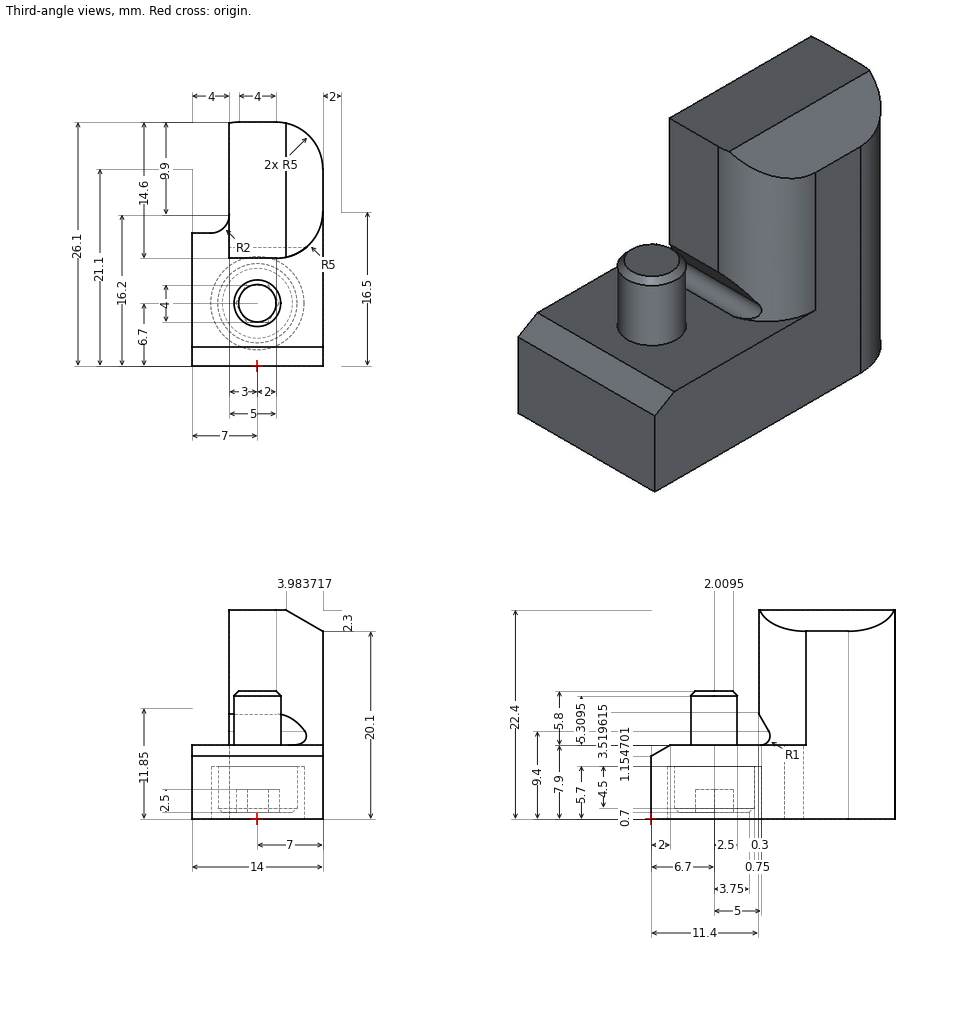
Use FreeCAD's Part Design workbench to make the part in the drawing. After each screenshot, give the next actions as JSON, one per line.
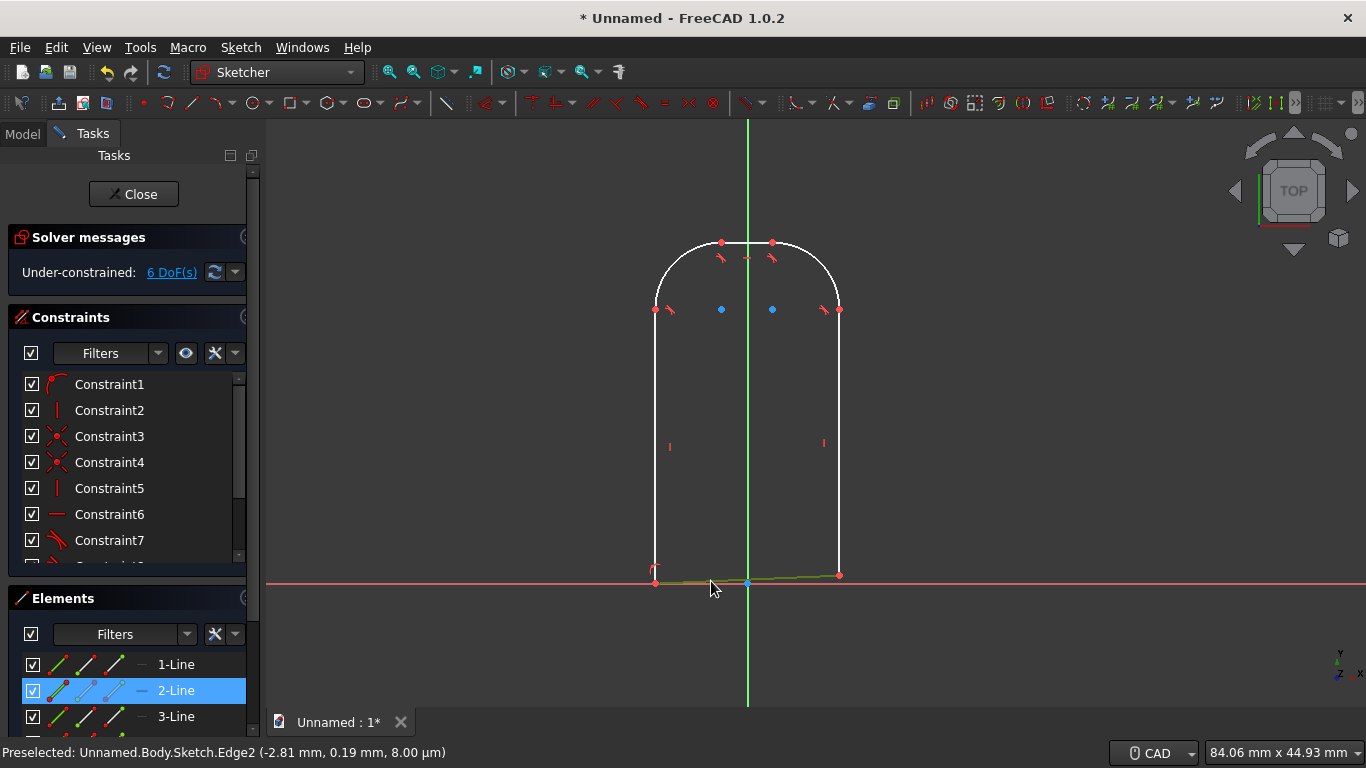
{"action": "key", "text": "h"}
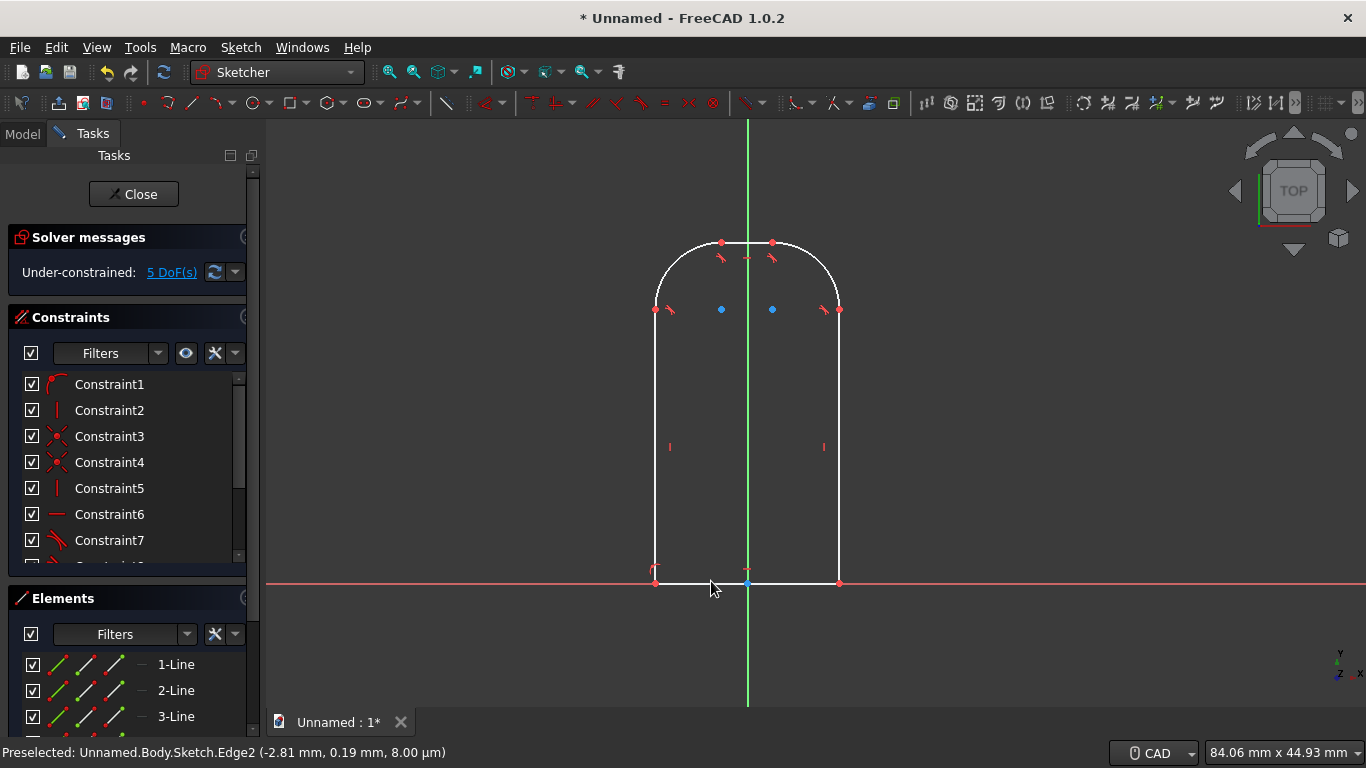
{"action": "left_click", "coordinate": [832, 279]}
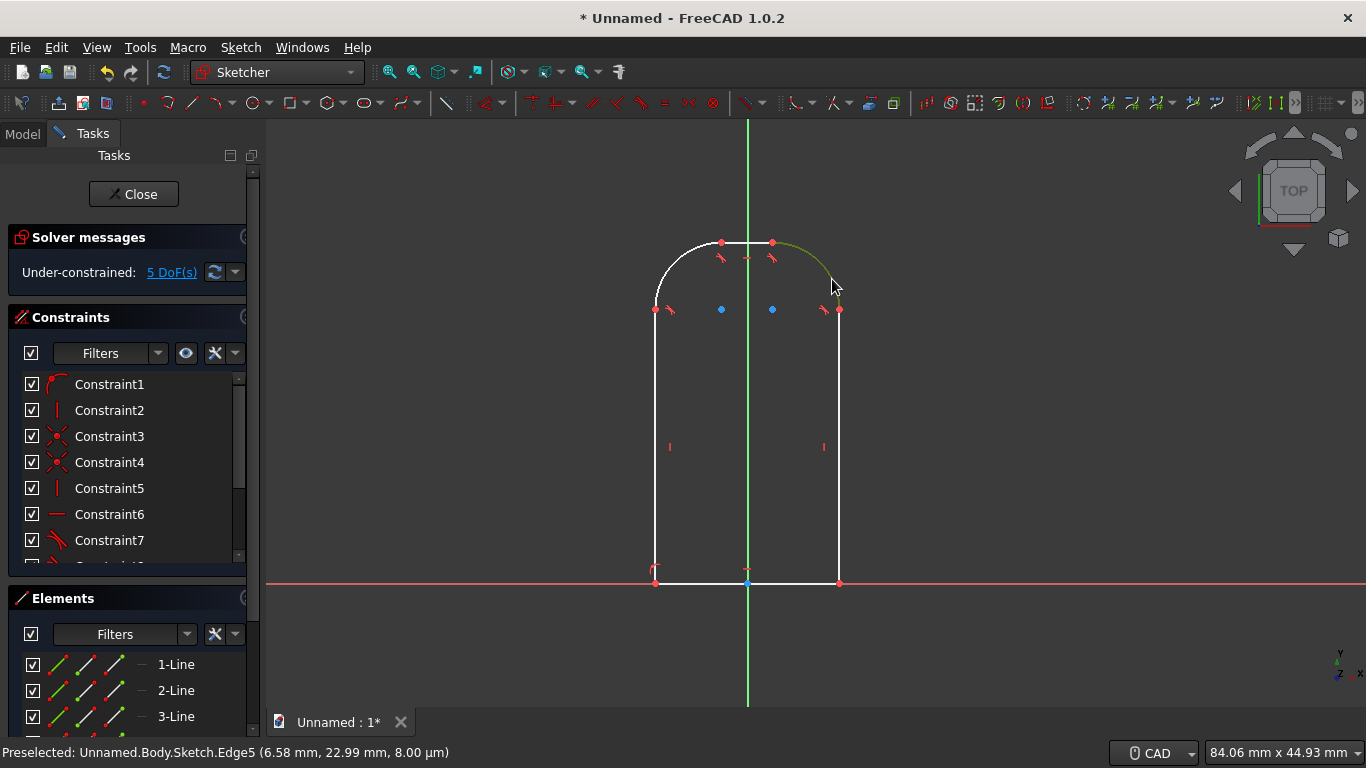
{"action": "left_click", "coordinate": [692, 250]}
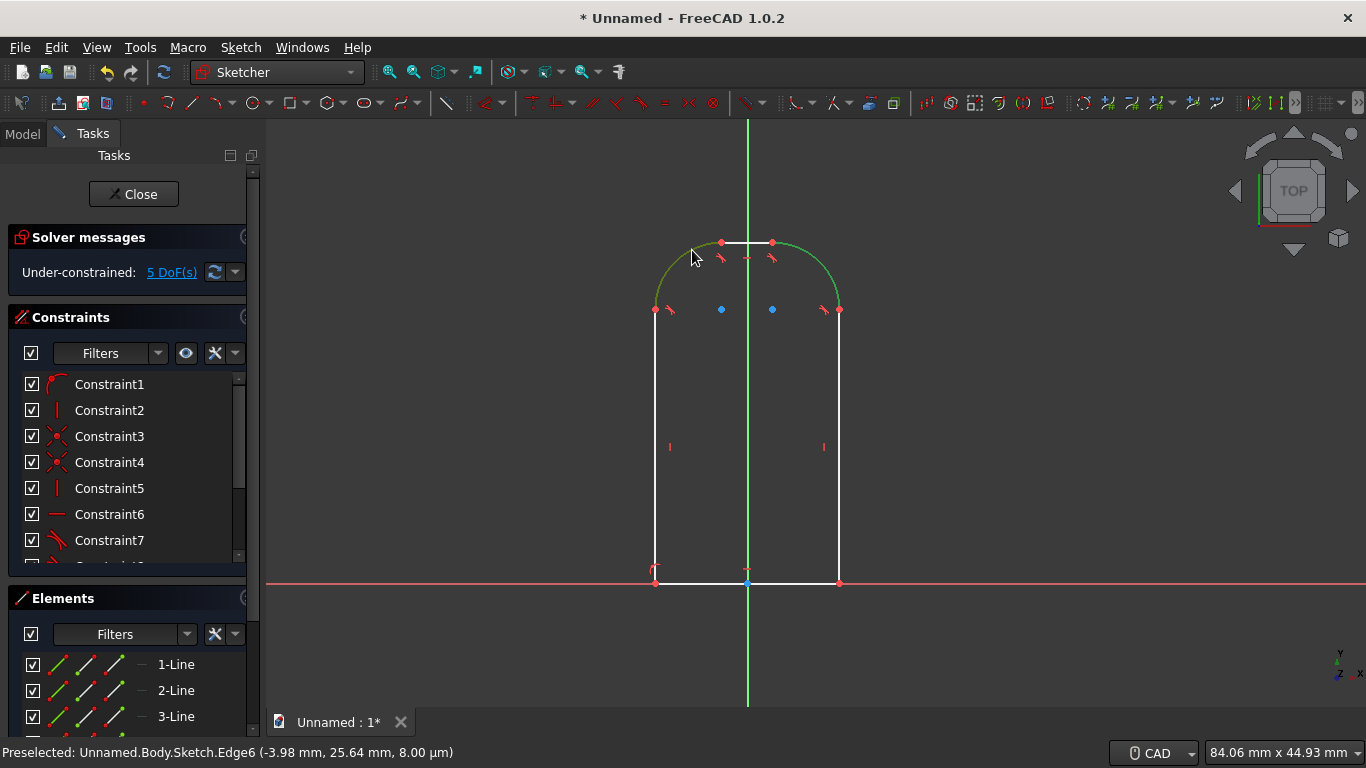
{"action": "left_click", "coordinate": [666, 104]}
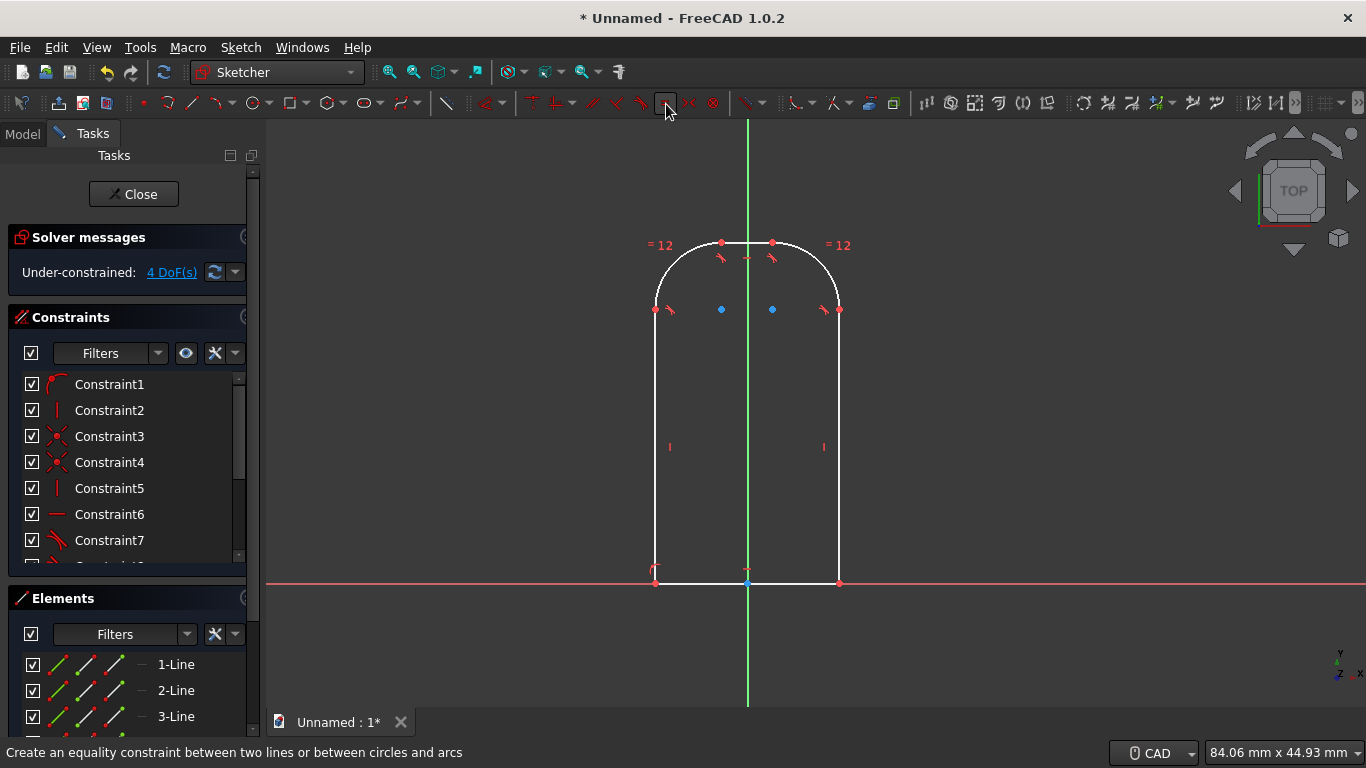
{"action": "left_click", "coordinate": [832, 279]}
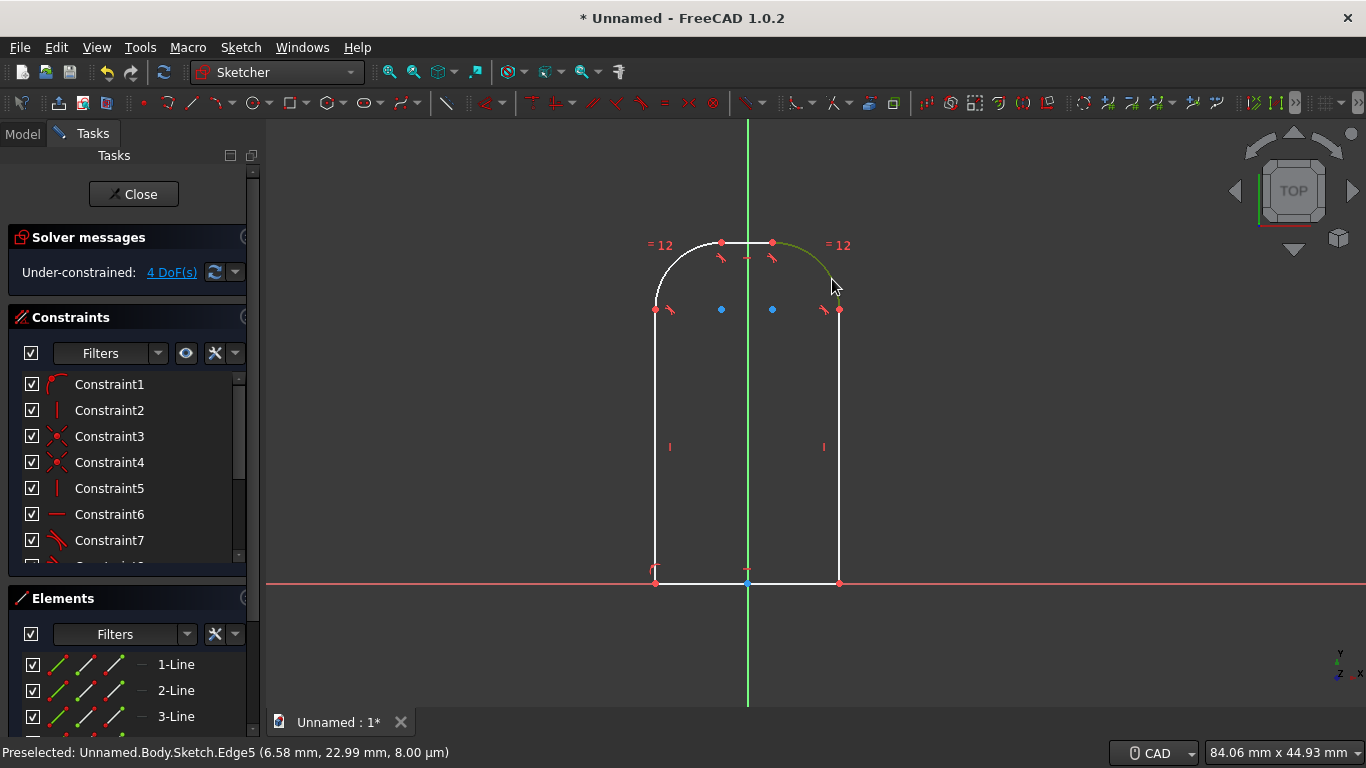
{"action": "key", "text": "k r"}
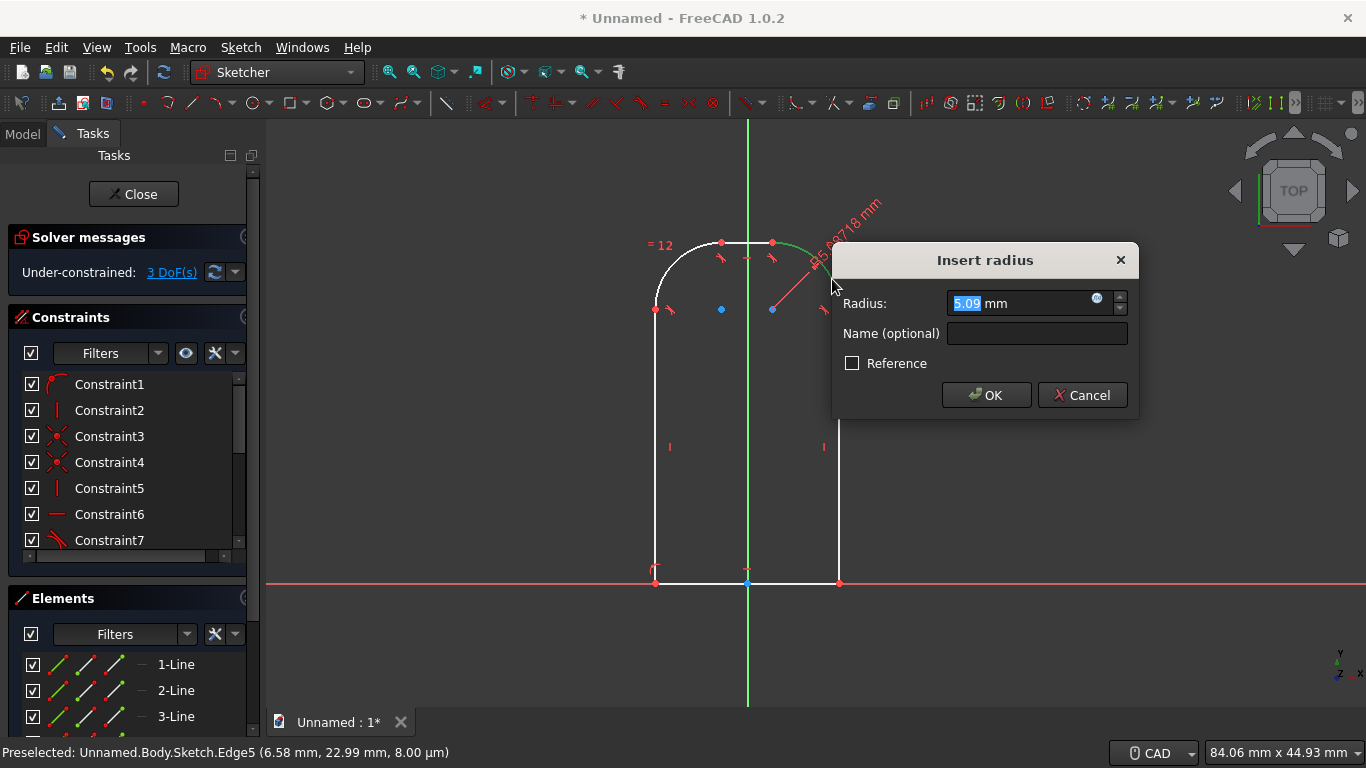
{"action": "type", "text": "5"}
{"action": "key", "text": "Return"}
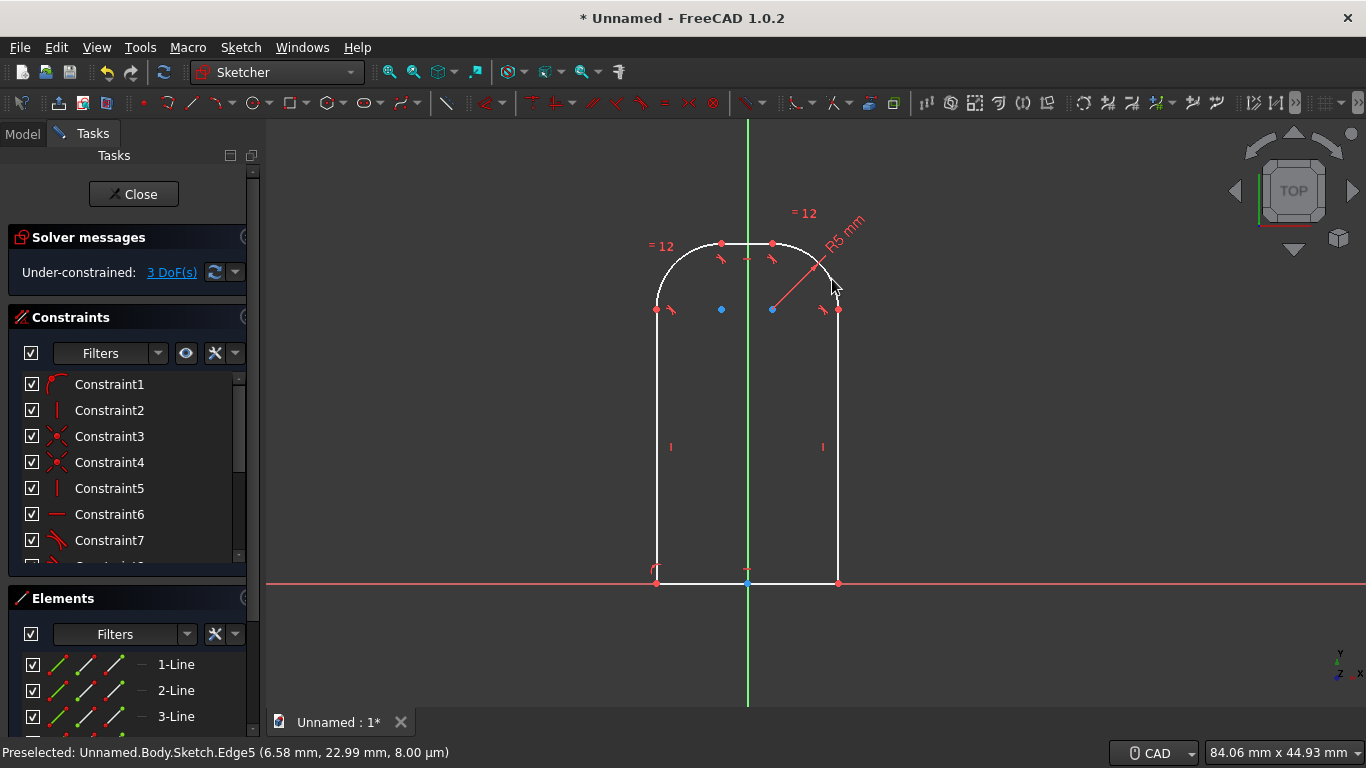
{"action": "scroll", "coordinate": [758, 244], "scroll_direction": "up", "scroll_amount": 2}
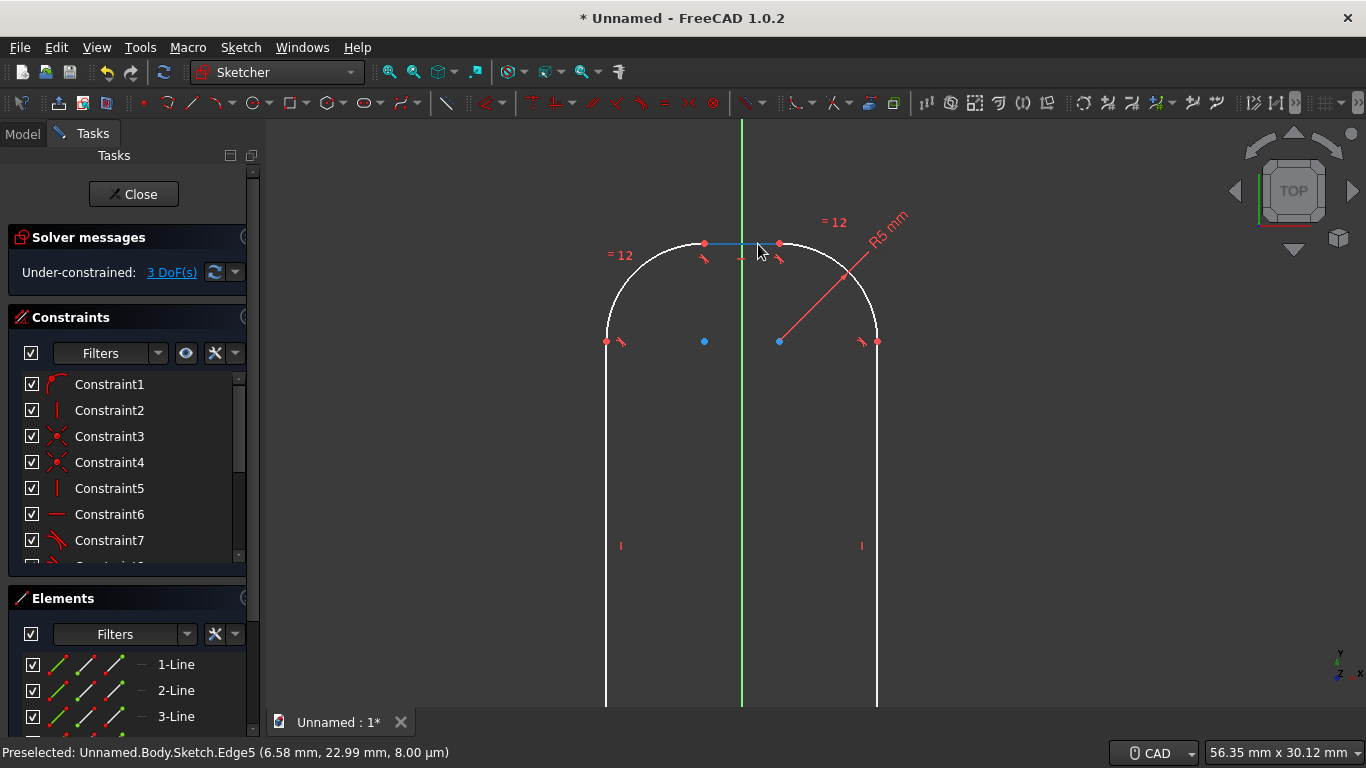
{"action": "left_click", "coordinate": [757, 244]}